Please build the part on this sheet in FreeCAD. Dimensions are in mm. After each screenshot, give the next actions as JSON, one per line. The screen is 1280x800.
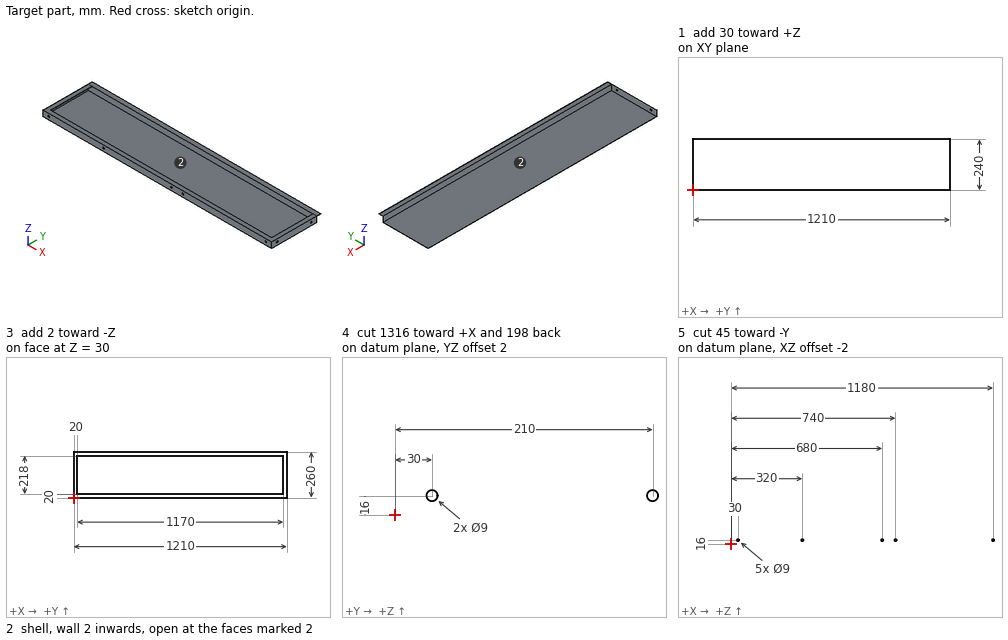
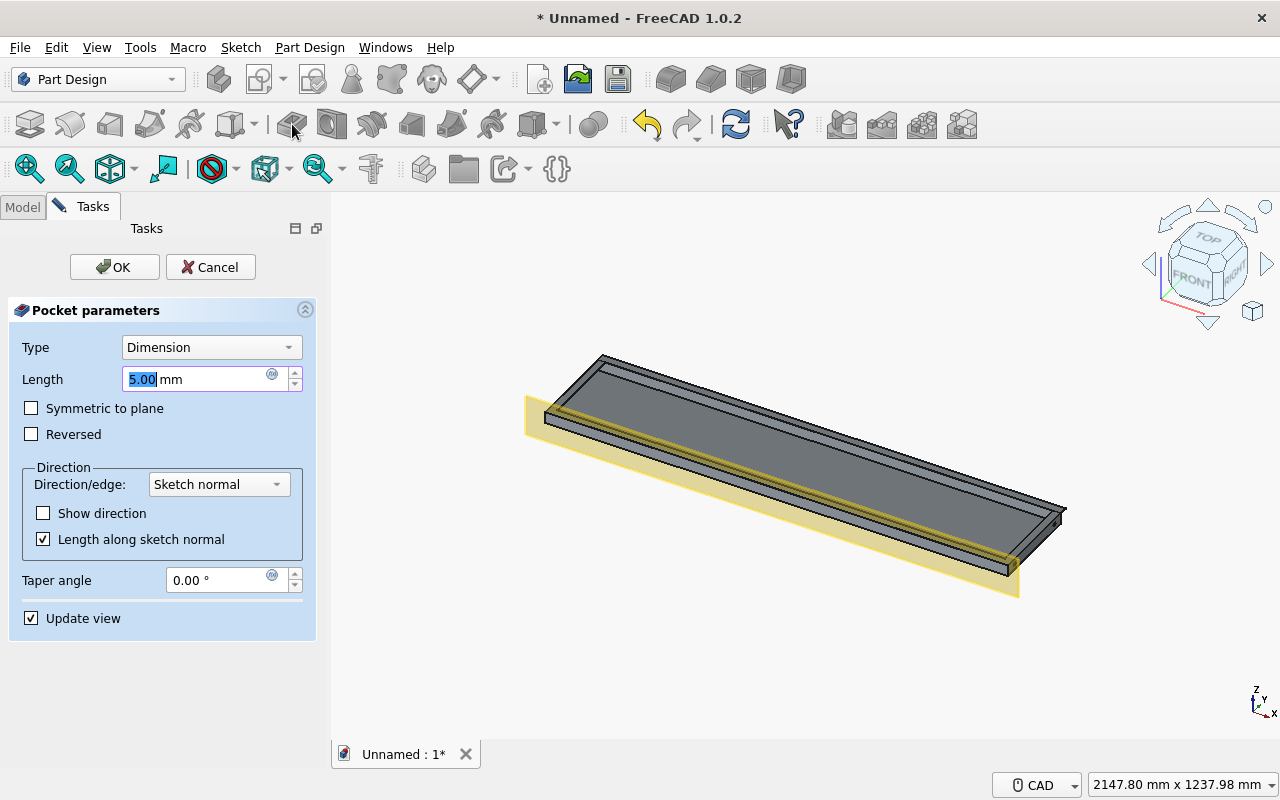
{"action": "type", "text": "45"}
{"action": "key", "text": "Tab"}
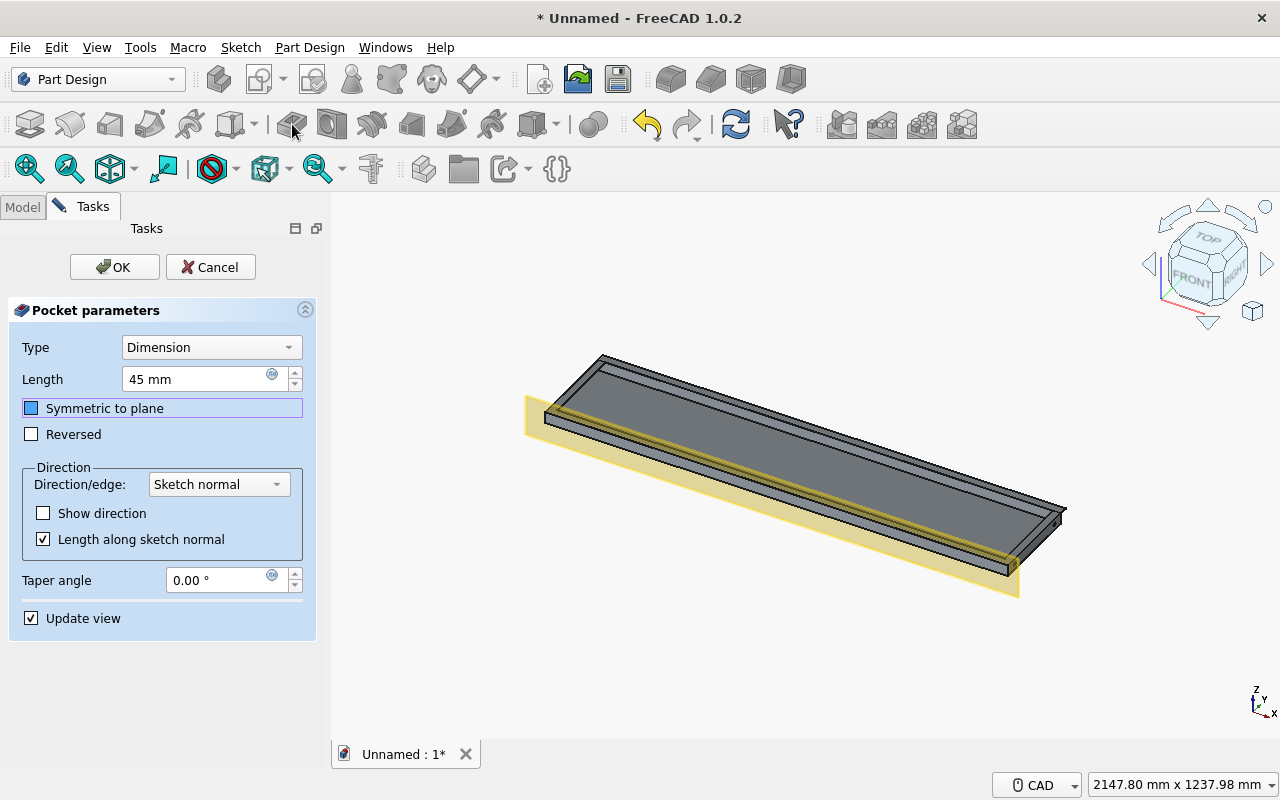
{"action": "left_click", "coordinate": [30, 434]}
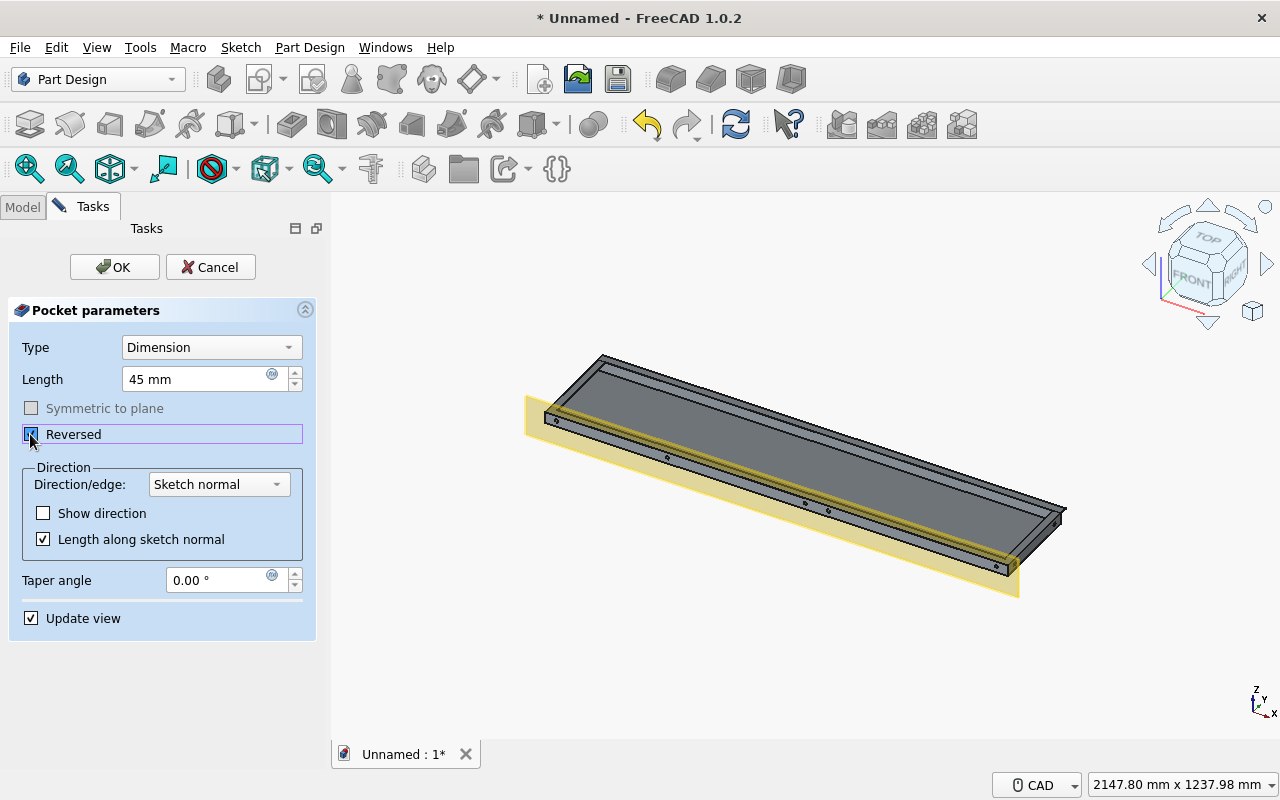
{"action": "left_click", "coordinate": [115, 267]}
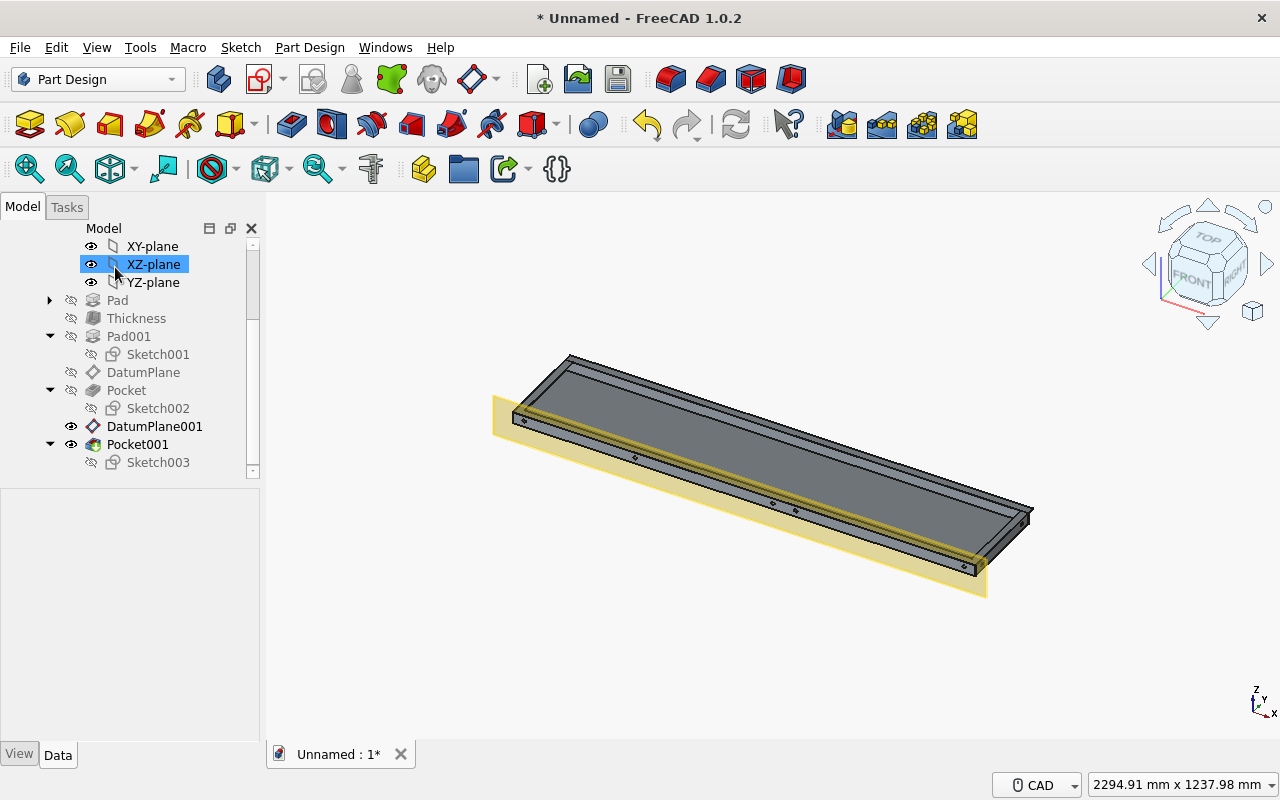
{"action": "left_click", "coordinate": [116, 426]}
{"action": "key", "text": "space"}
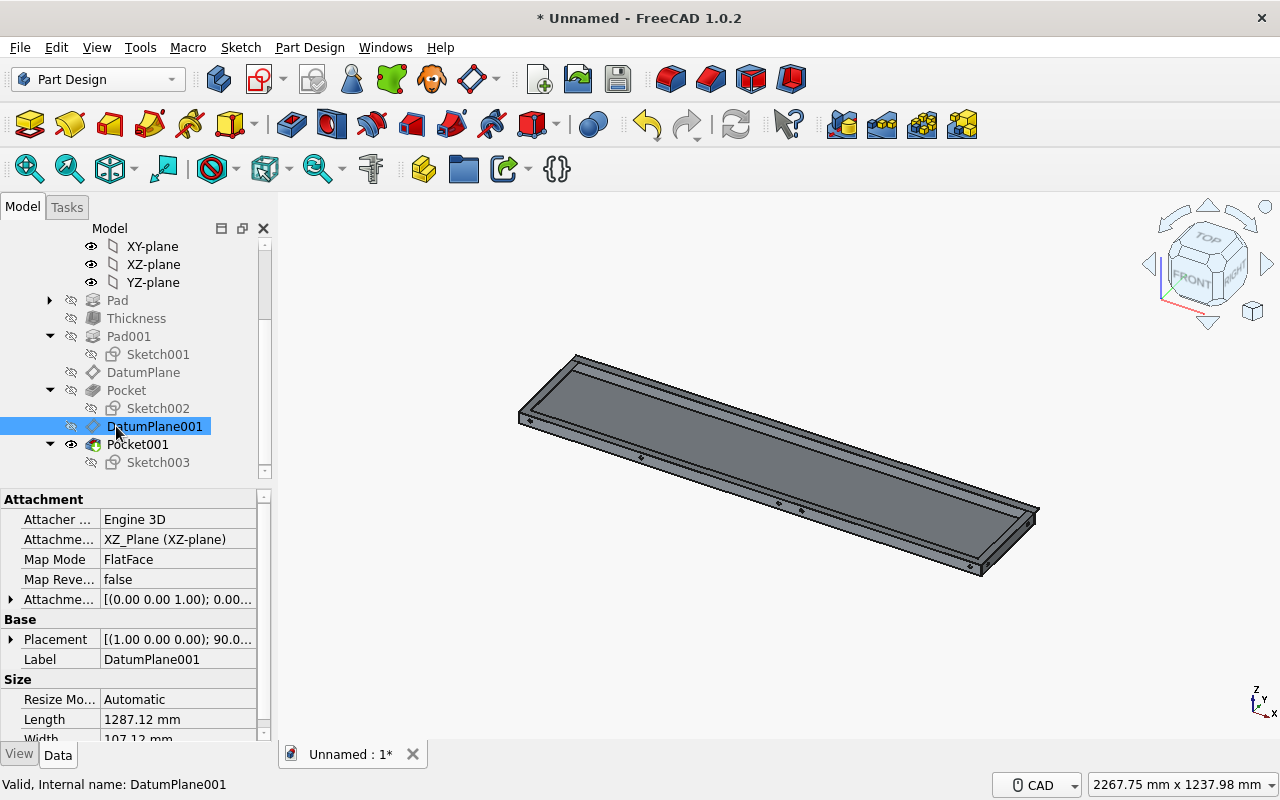
{"action": "key", "text": "0"}